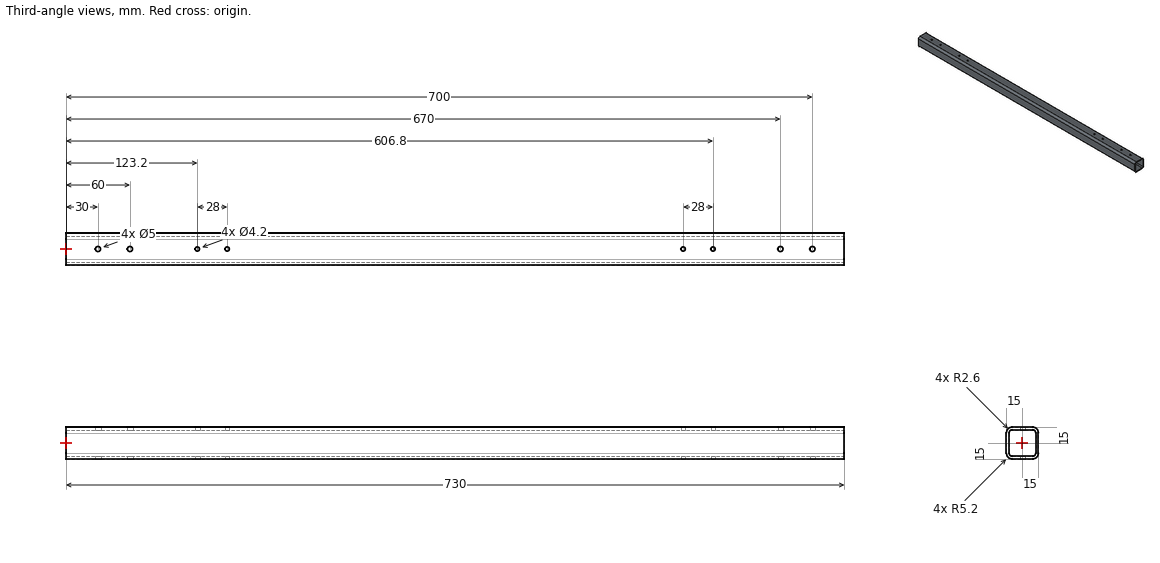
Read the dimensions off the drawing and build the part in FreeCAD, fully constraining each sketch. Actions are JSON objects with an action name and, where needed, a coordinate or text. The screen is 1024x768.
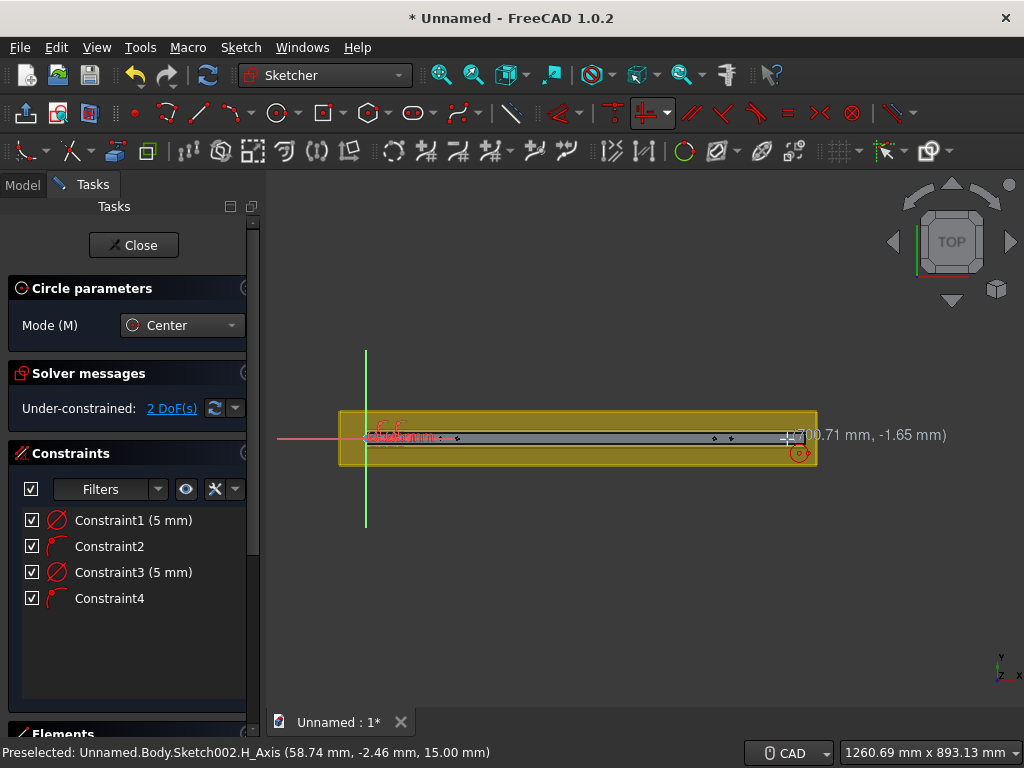
{"action": "left_click", "coordinate": [787, 439]}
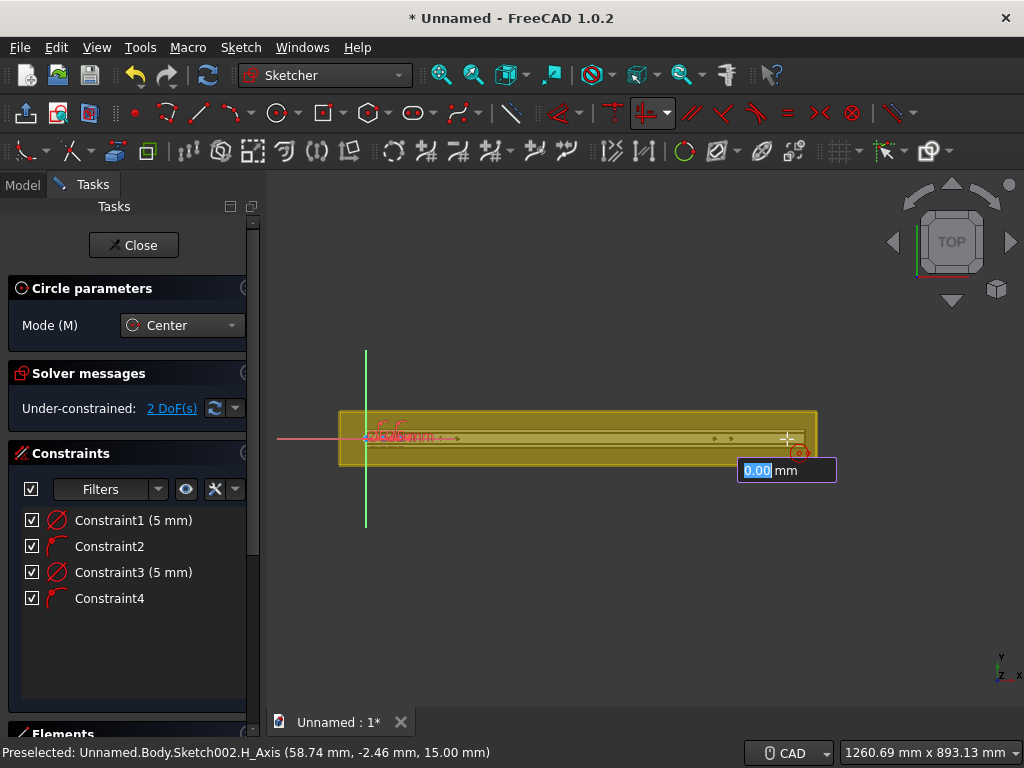
{"action": "scroll", "coordinate": [787, 440], "scroll_direction": "up", "scroll_amount": 13}
{"action": "mouse_move", "coordinate": [774, 433]}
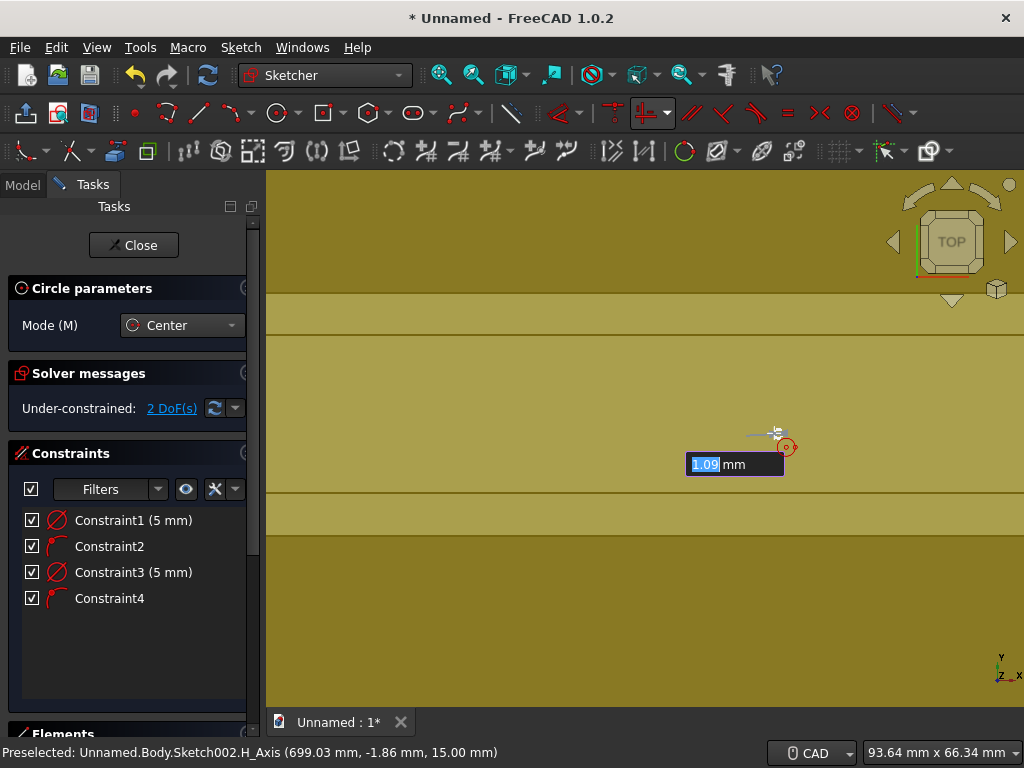
{"action": "type", "text": "5"}
{"action": "key", "text": "Return"}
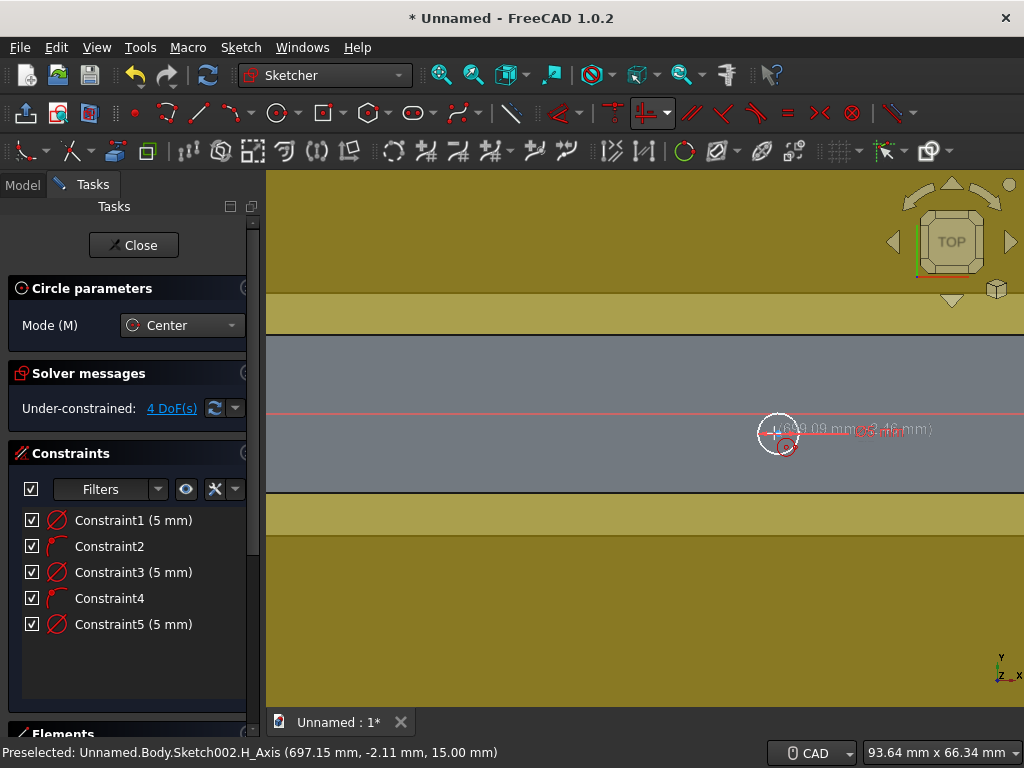
{"action": "scroll", "coordinate": [787, 440], "scroll_direction": "down", "scroll_amount": 13}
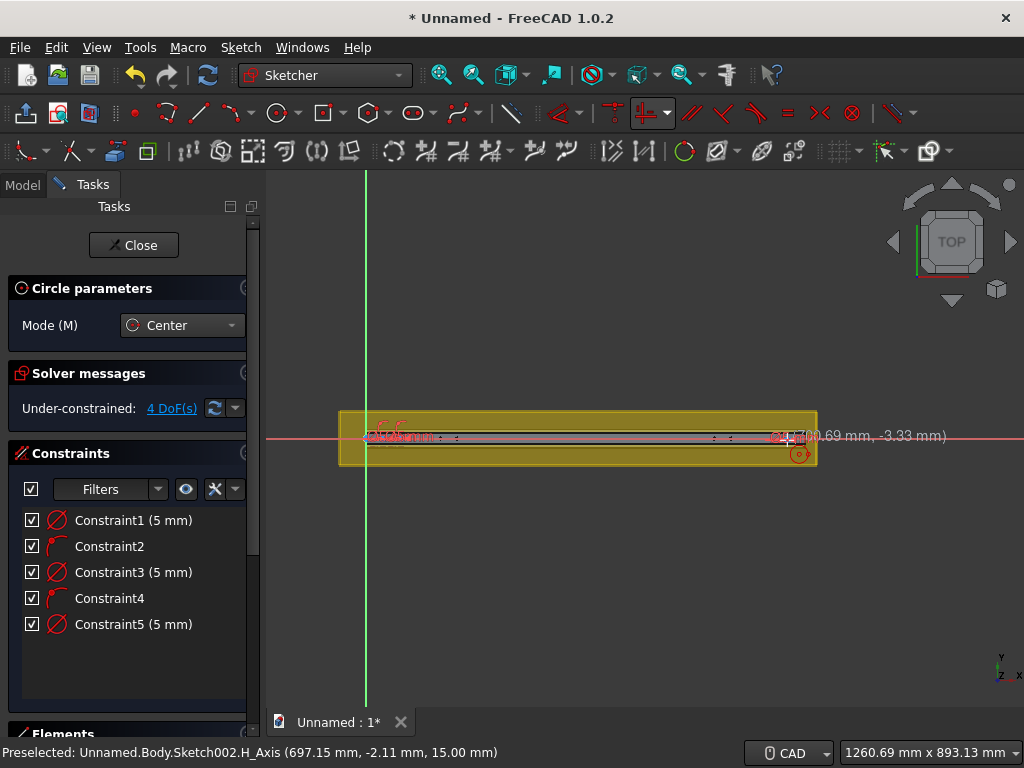
{"action": "left_click", "coordinate": [769, 439]}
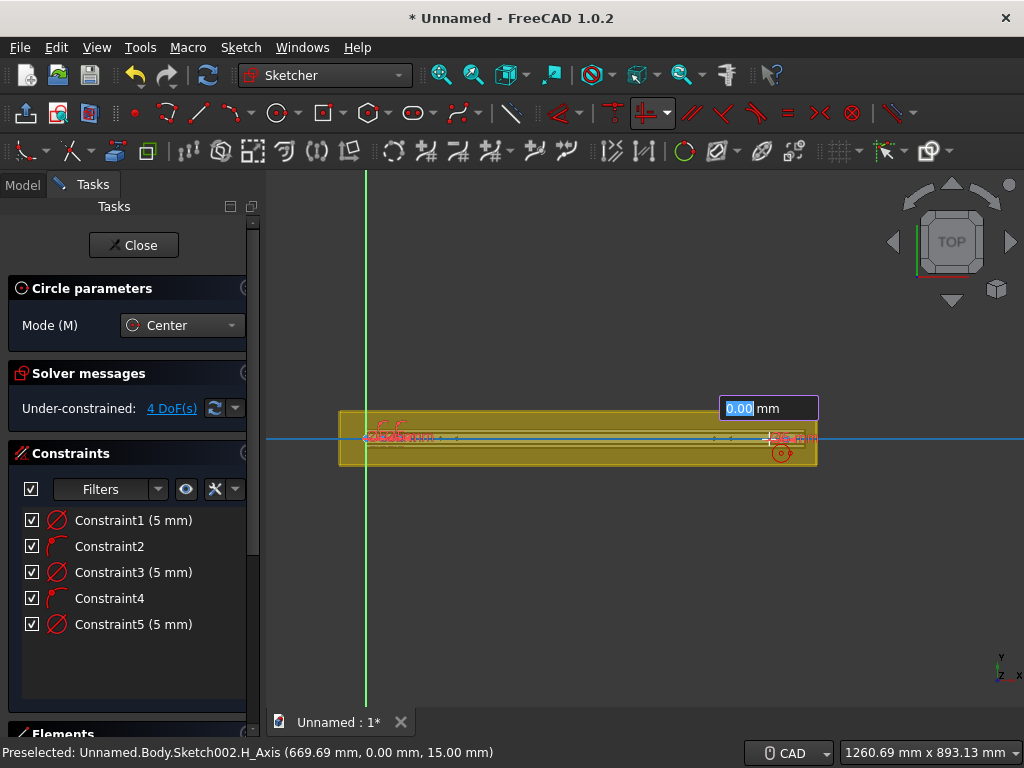
{"action": "scroll", "coordinate": [769, 440], "scroll_direction": "up", "scroll_amount": 13}
{"action": "mouse_move", "coordinate": [756, 433]}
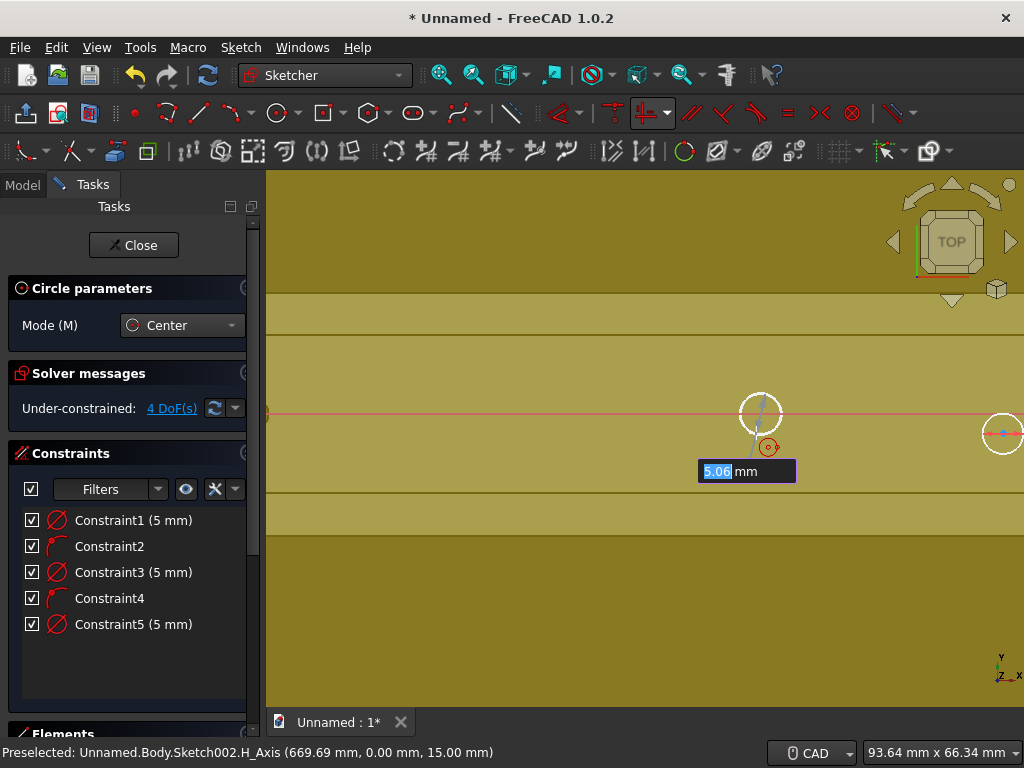
{"action": "type", "text": "5"}
{"action": "key", "text": "Return"}
{"action": "key", "text": "Escape"}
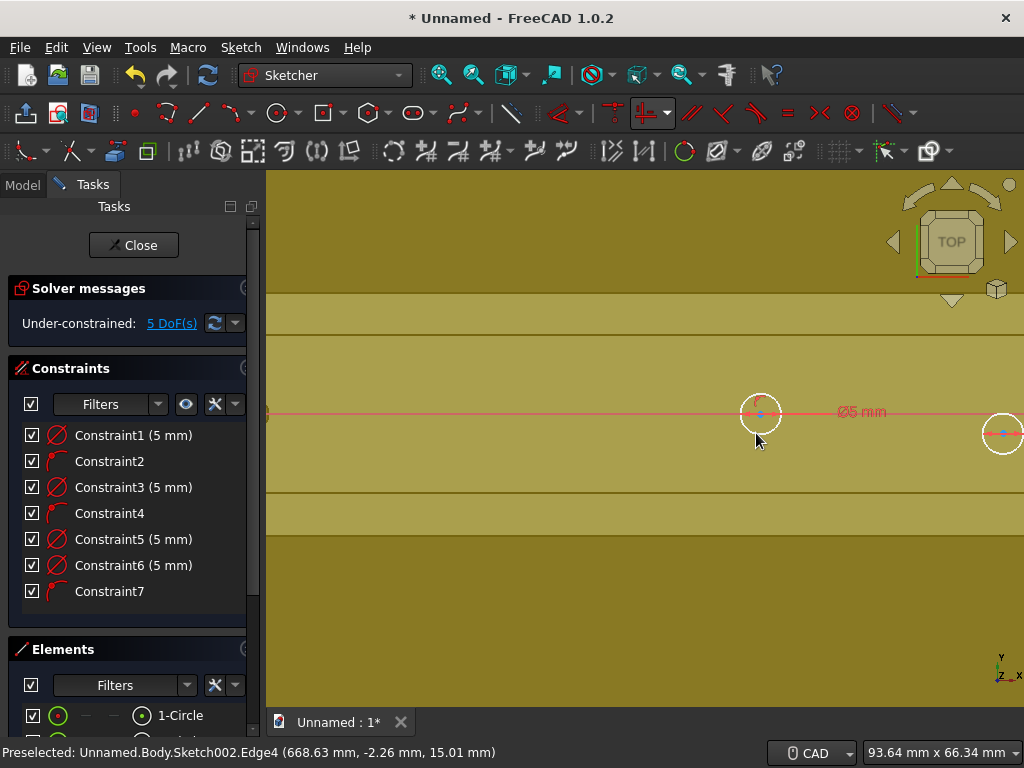
{"action": "scroll", "coordinate": [769, 440], "scroll_direction": "down", "scroll_amount": 13}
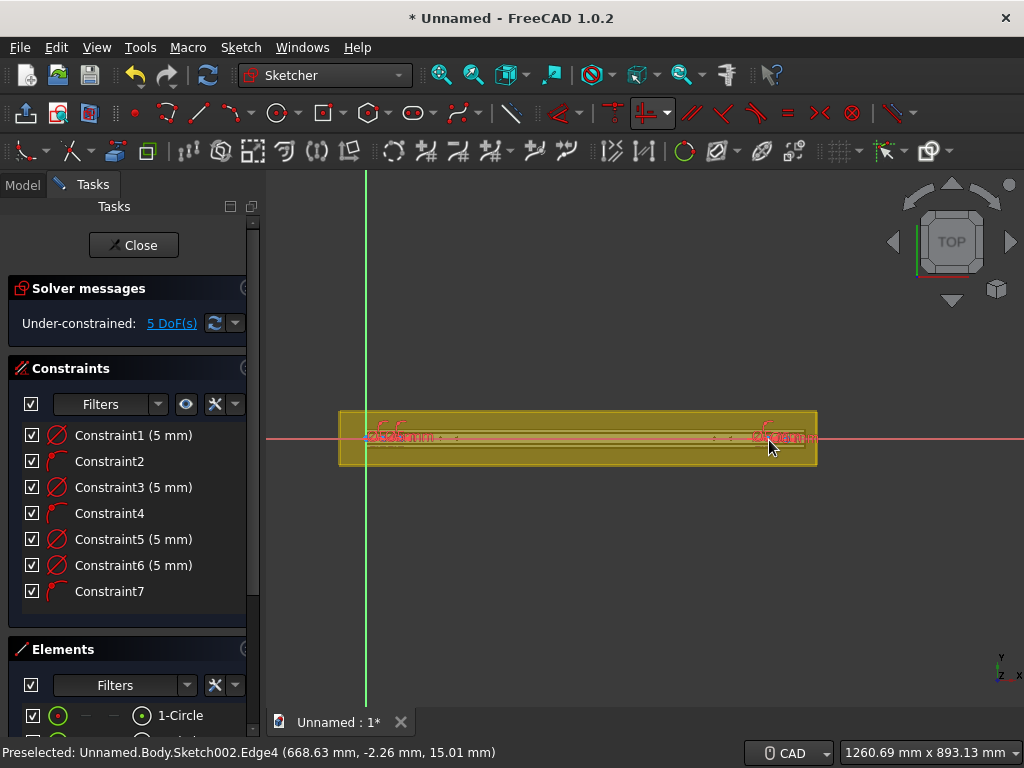
{"action": "left_click", "coordinate": [787, 440]}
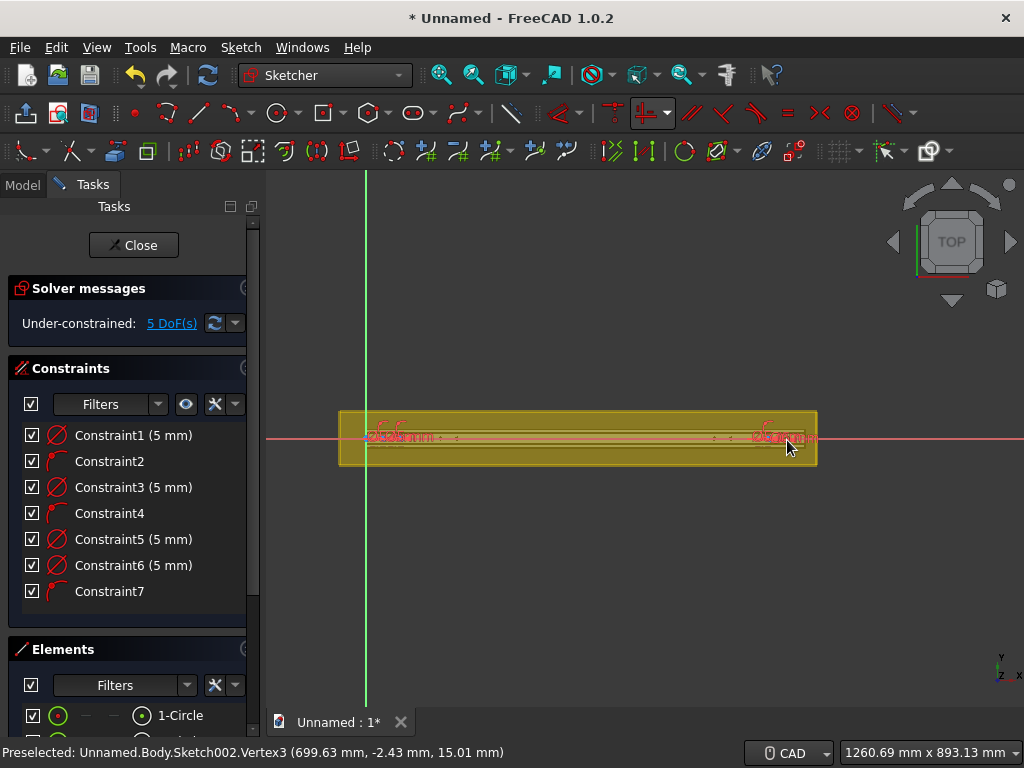
{"action": "left_click", "coordinate": [334, 439]}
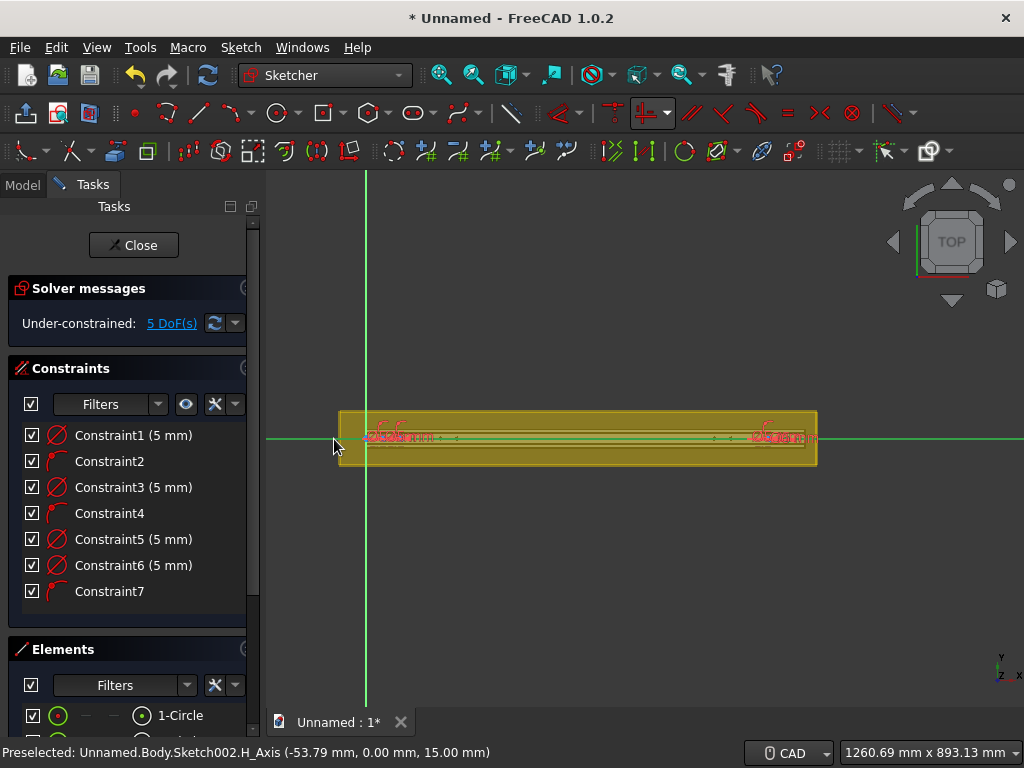
{"action": "left_click", "coordinate": [614, 114]}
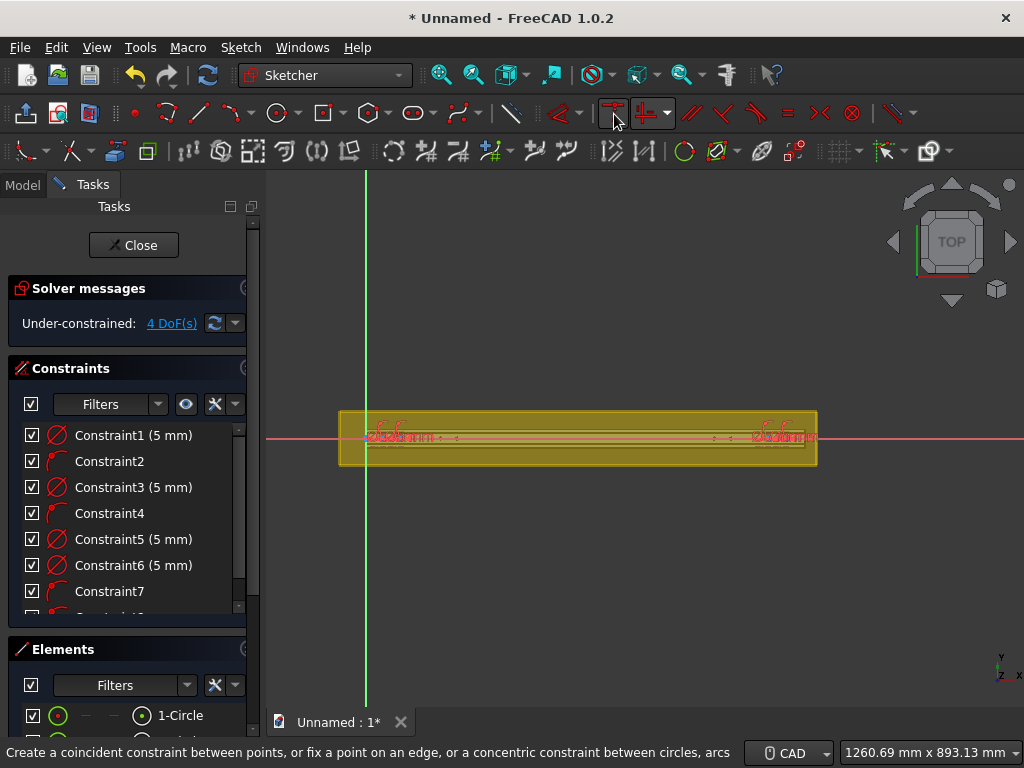
{"action": "left_click", "coordinate": [558, 114]}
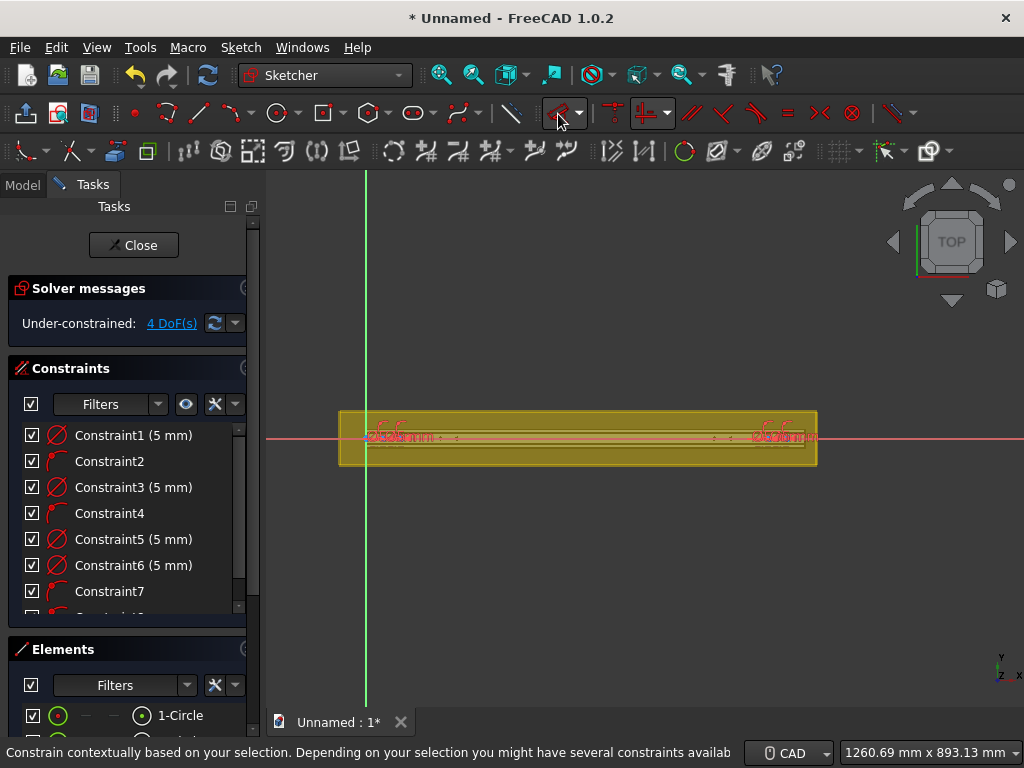
{"action": "scroll", "coordinate": [384, 439], "scroll_direction": "up", "scroll_amount": 4}